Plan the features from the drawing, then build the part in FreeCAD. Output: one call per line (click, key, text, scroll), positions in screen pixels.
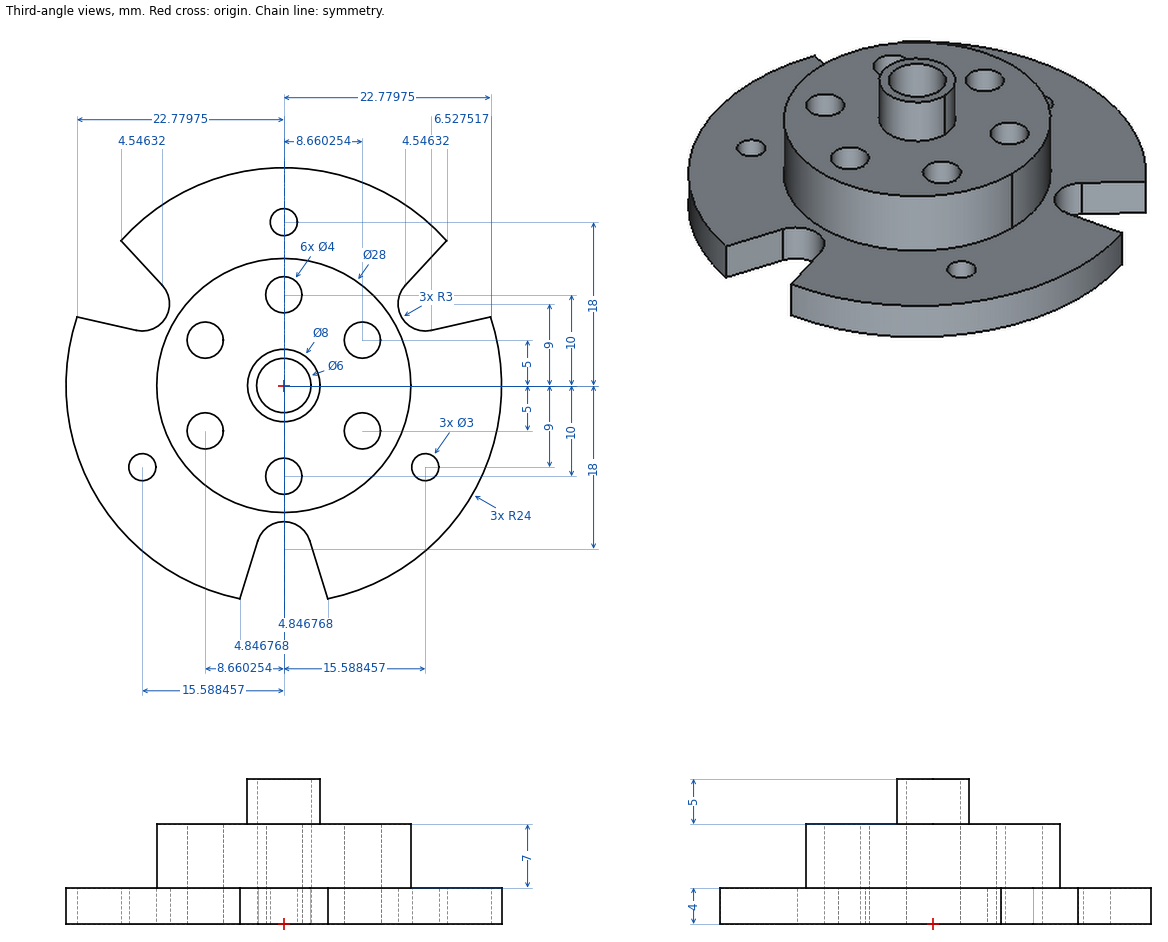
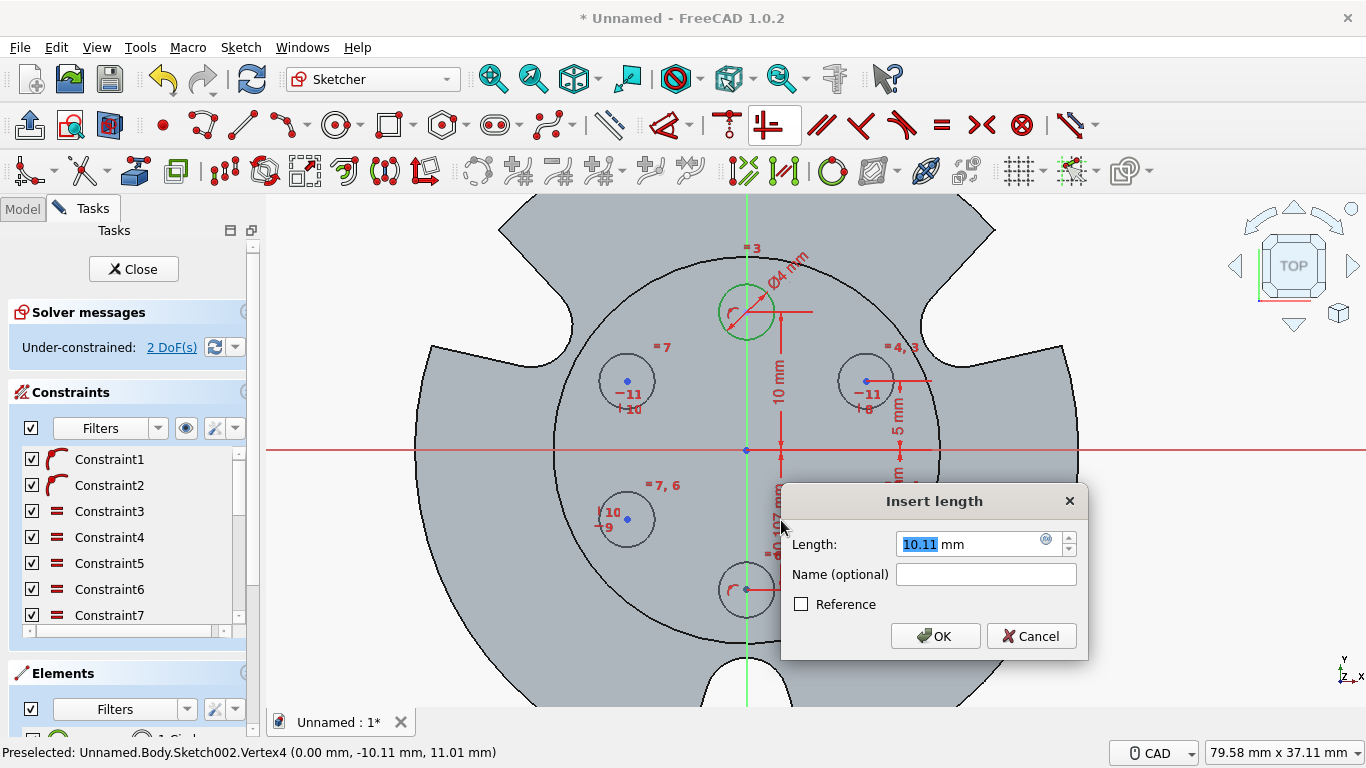
text(10)
key(Return)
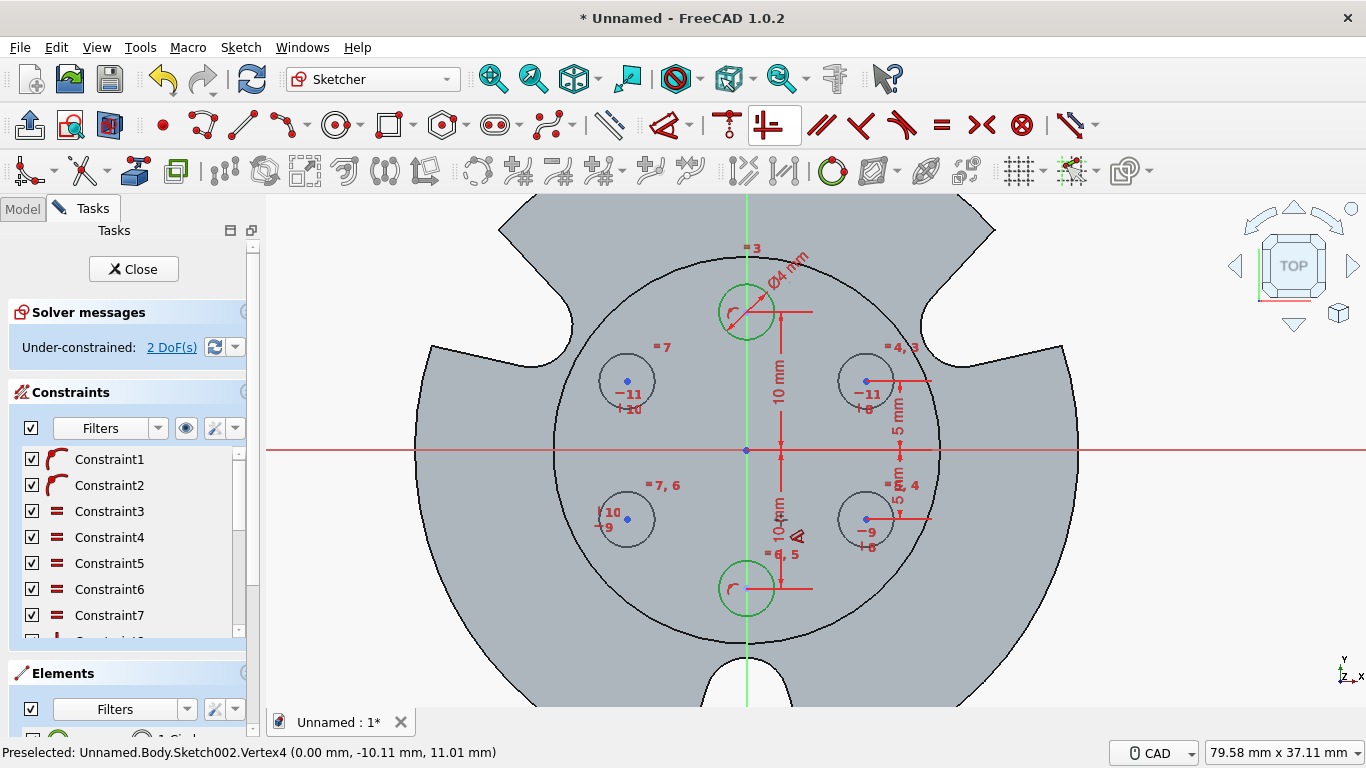
click(866, 381)
click(806, 347)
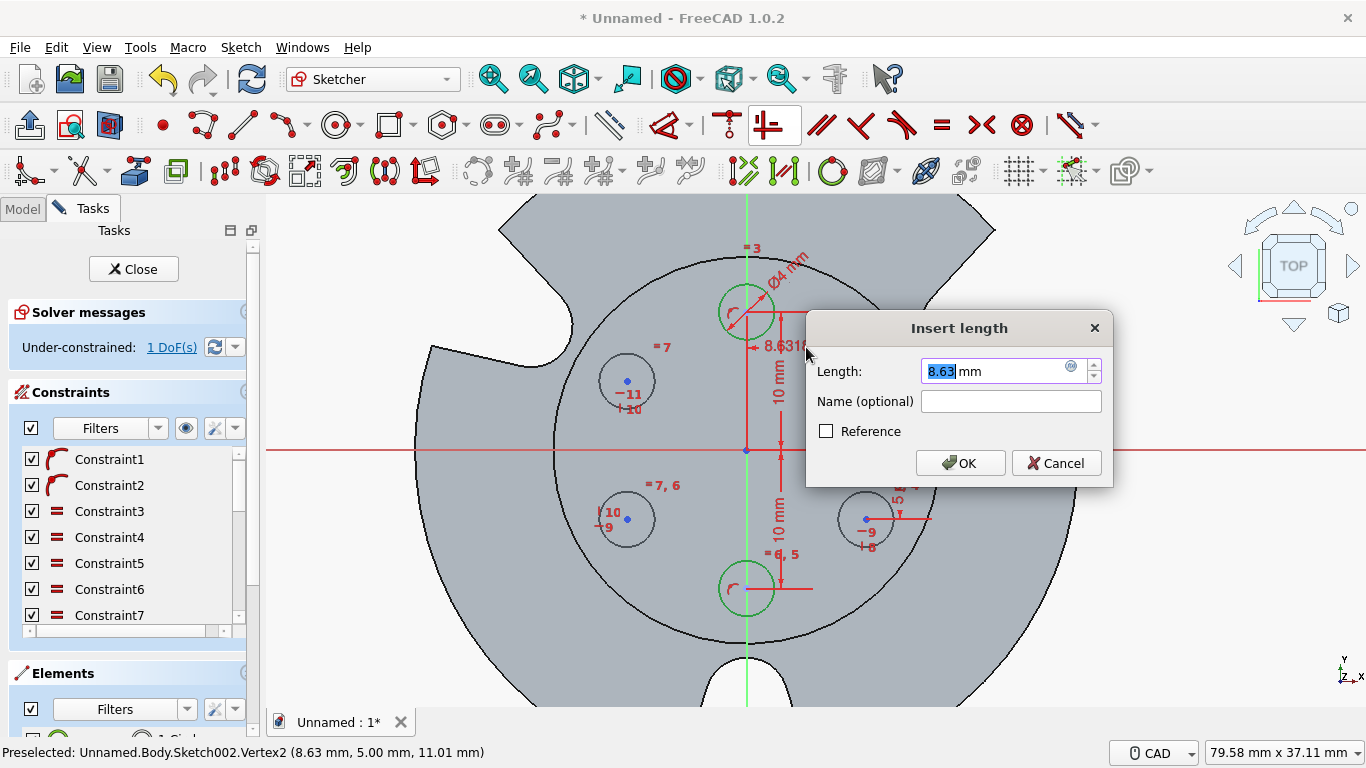
text(8.660254)
key(Return)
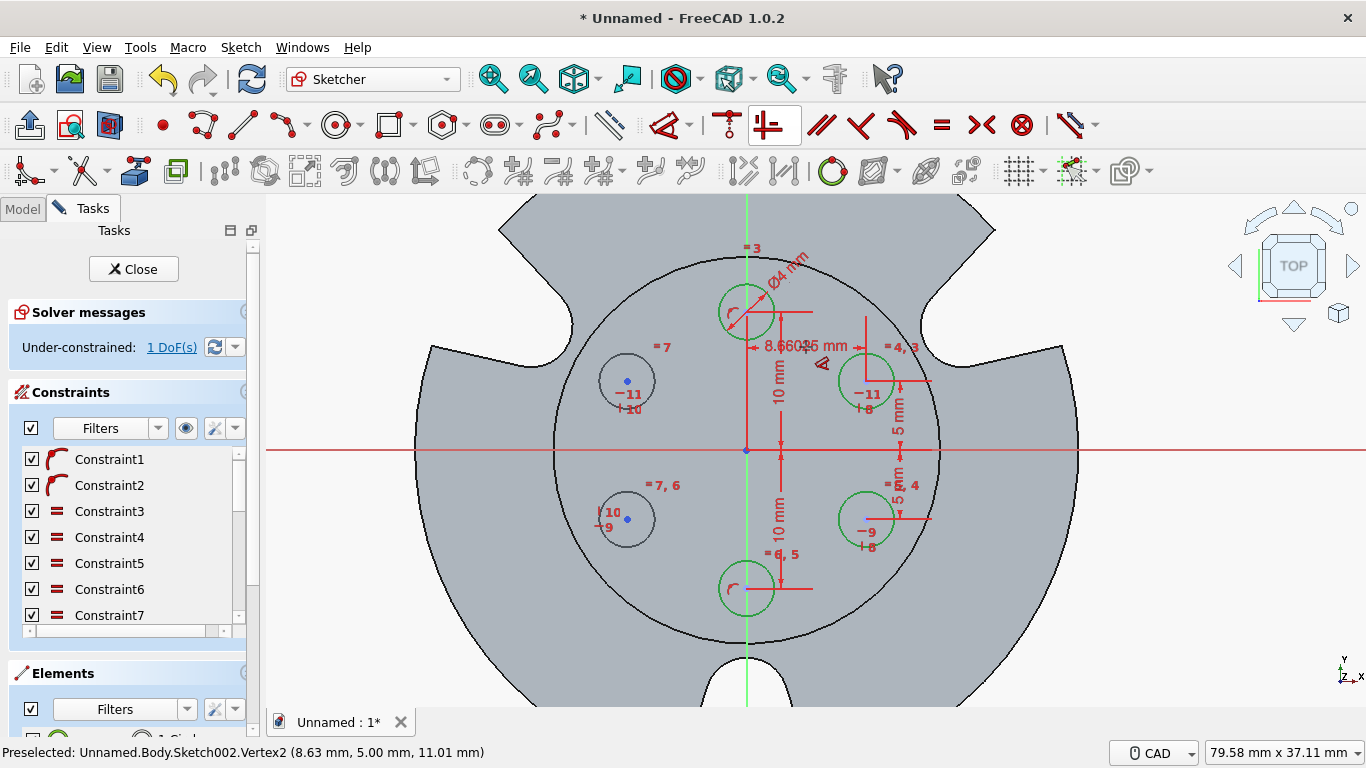
click(627, 519)
click(687, 553)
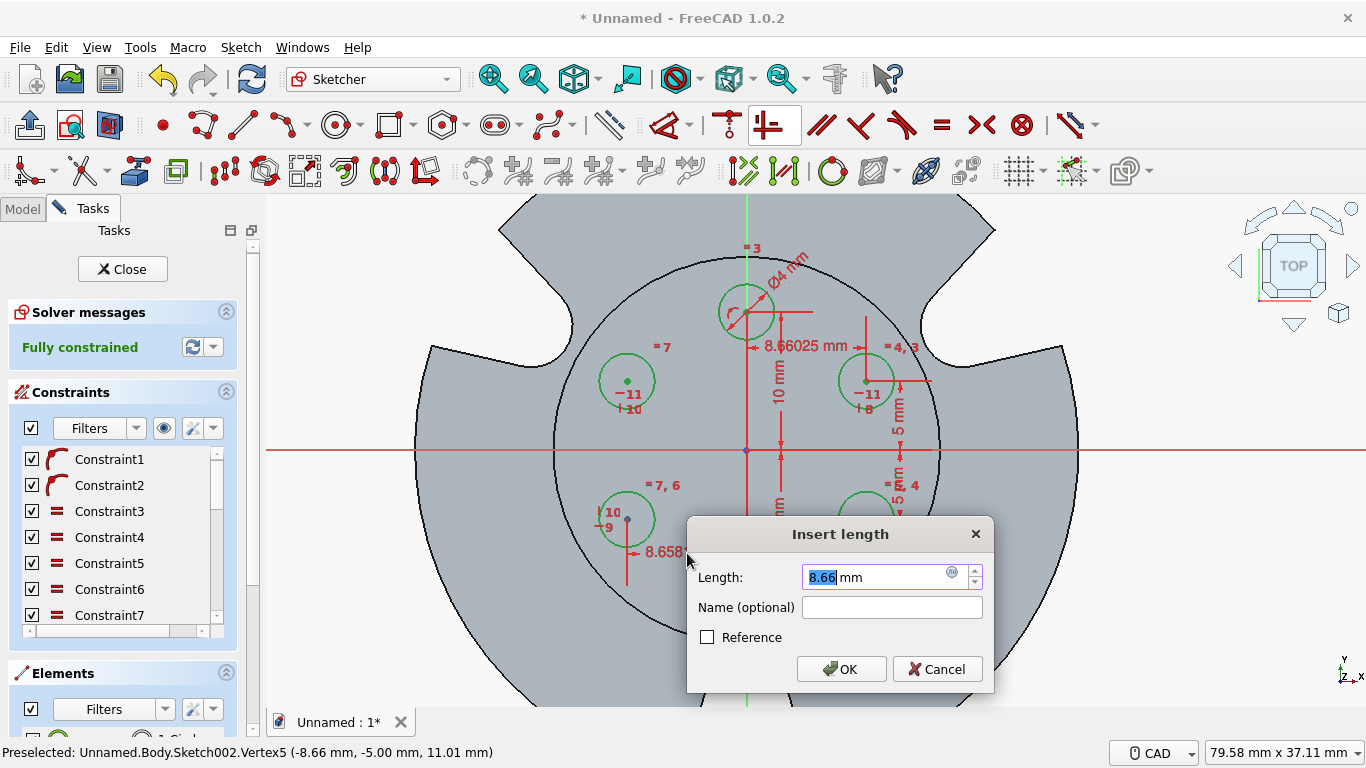
text(8.660254)
key(Return)
key(Escape)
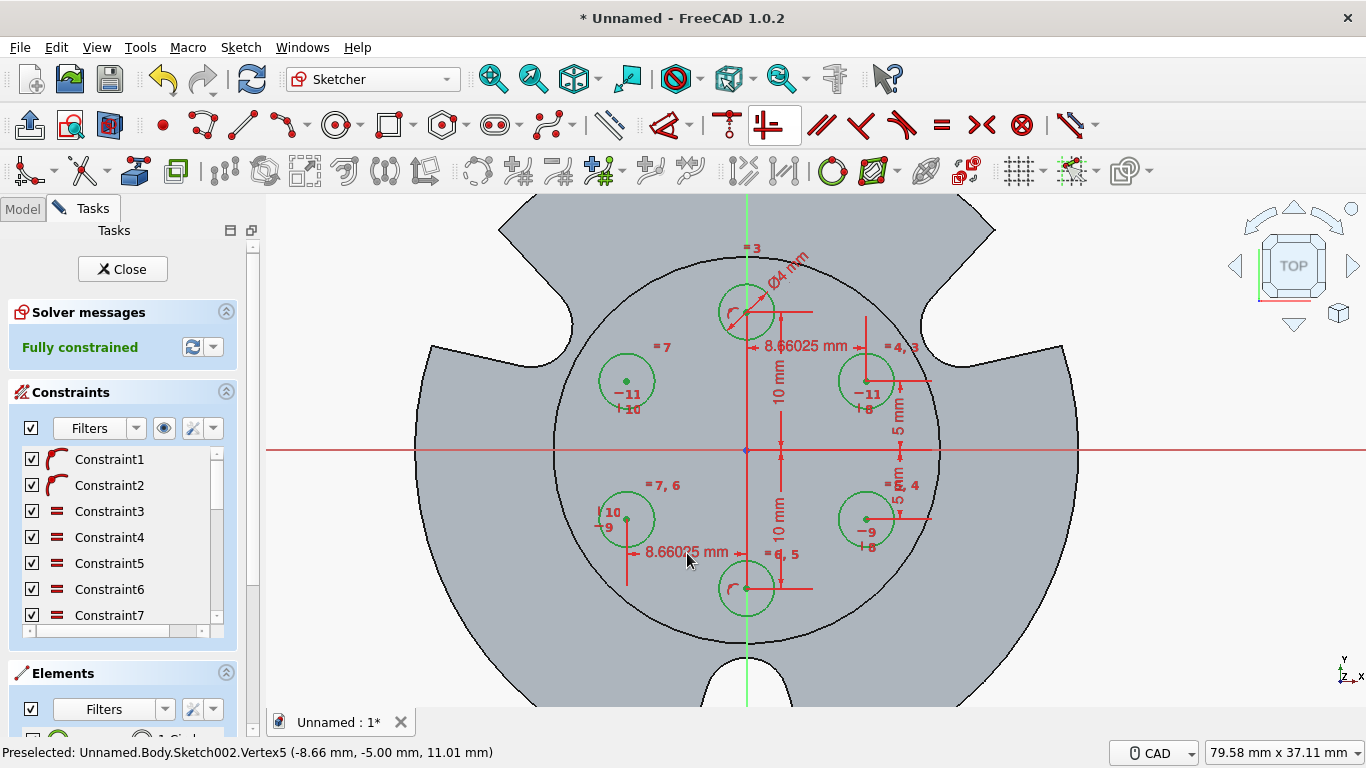
click(123, 269)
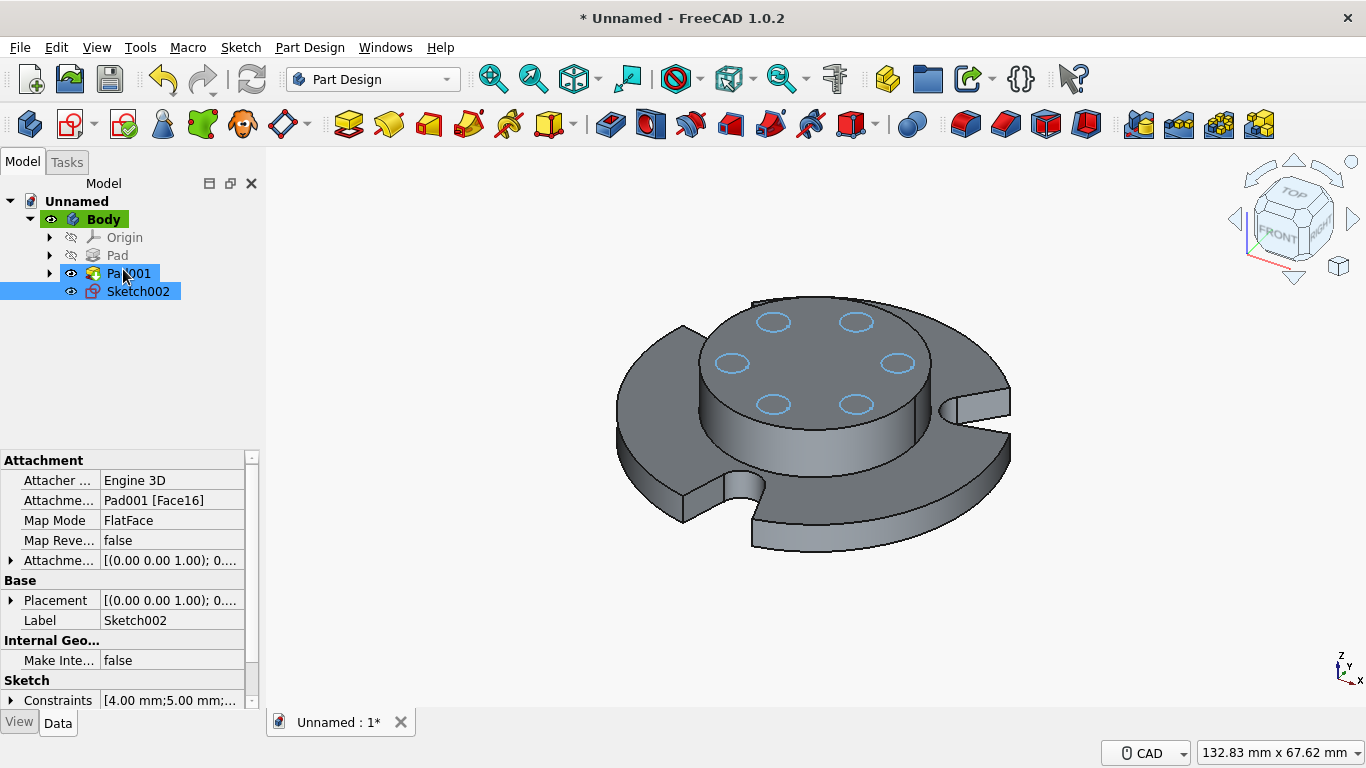
click(612, 124)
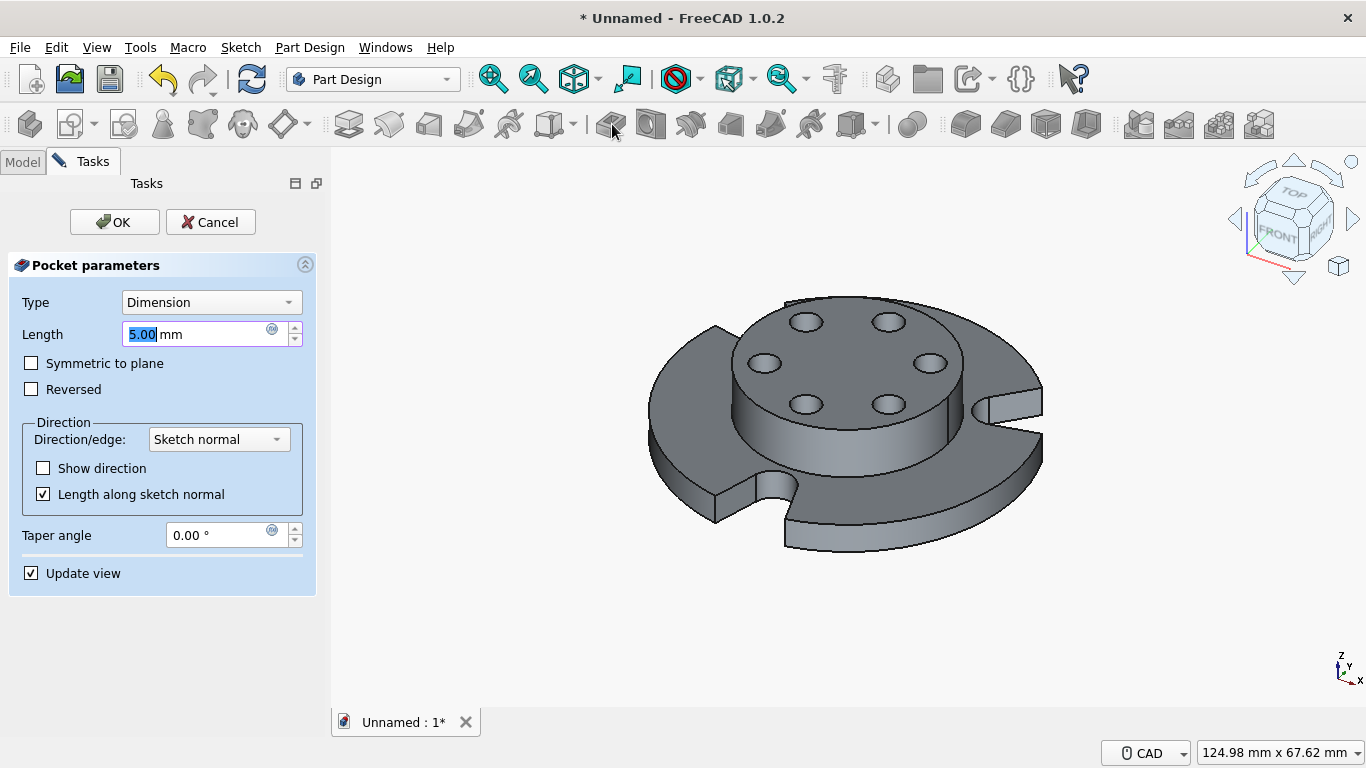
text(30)
key(Tab)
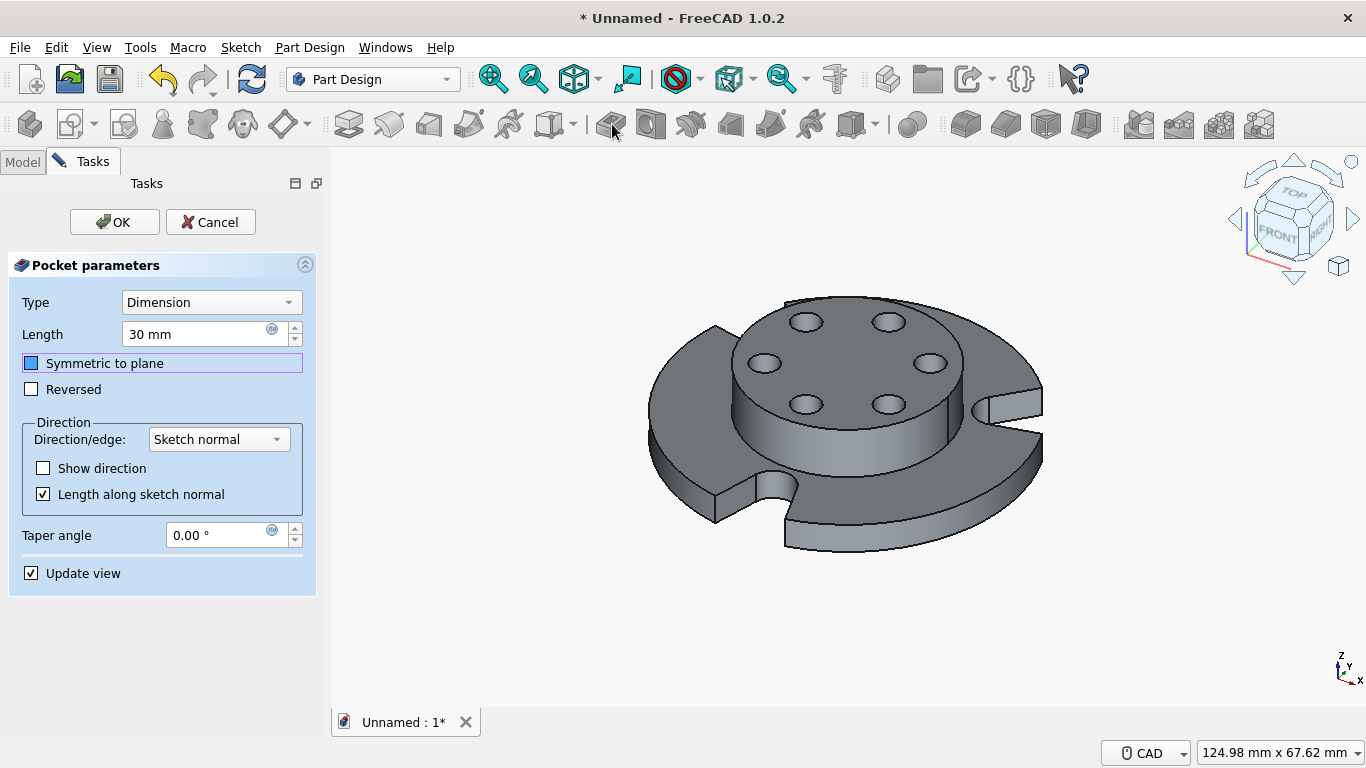
click(115, 222)